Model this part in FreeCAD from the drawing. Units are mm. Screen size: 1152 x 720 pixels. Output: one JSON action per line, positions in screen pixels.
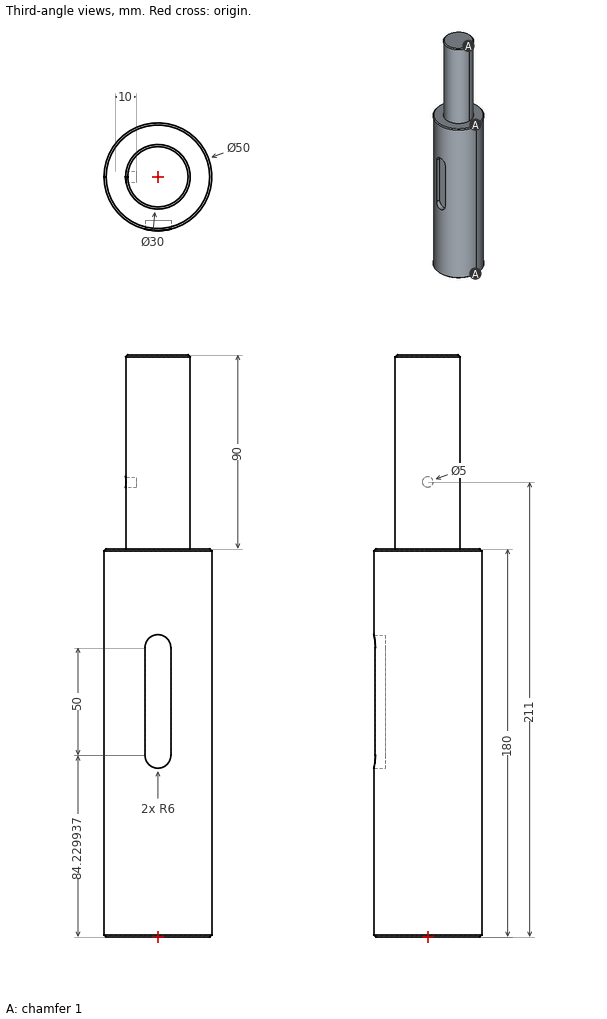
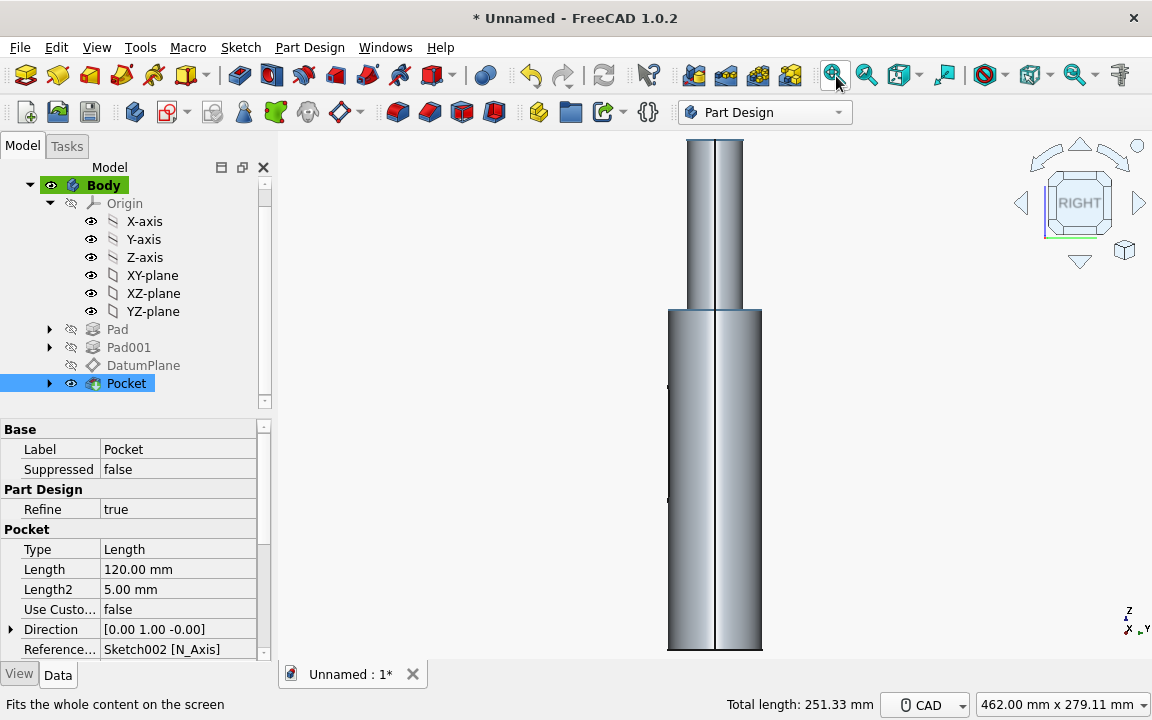
{"action": "key", "text": "5"}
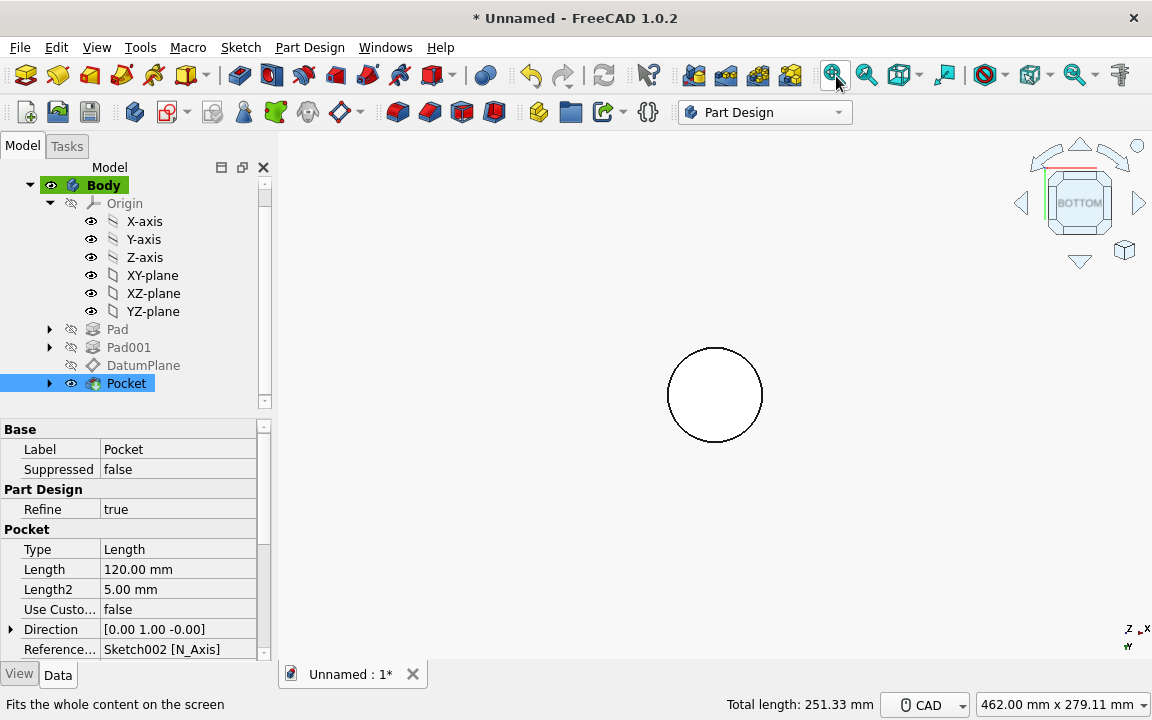
{"action": "key", "text": "v f"}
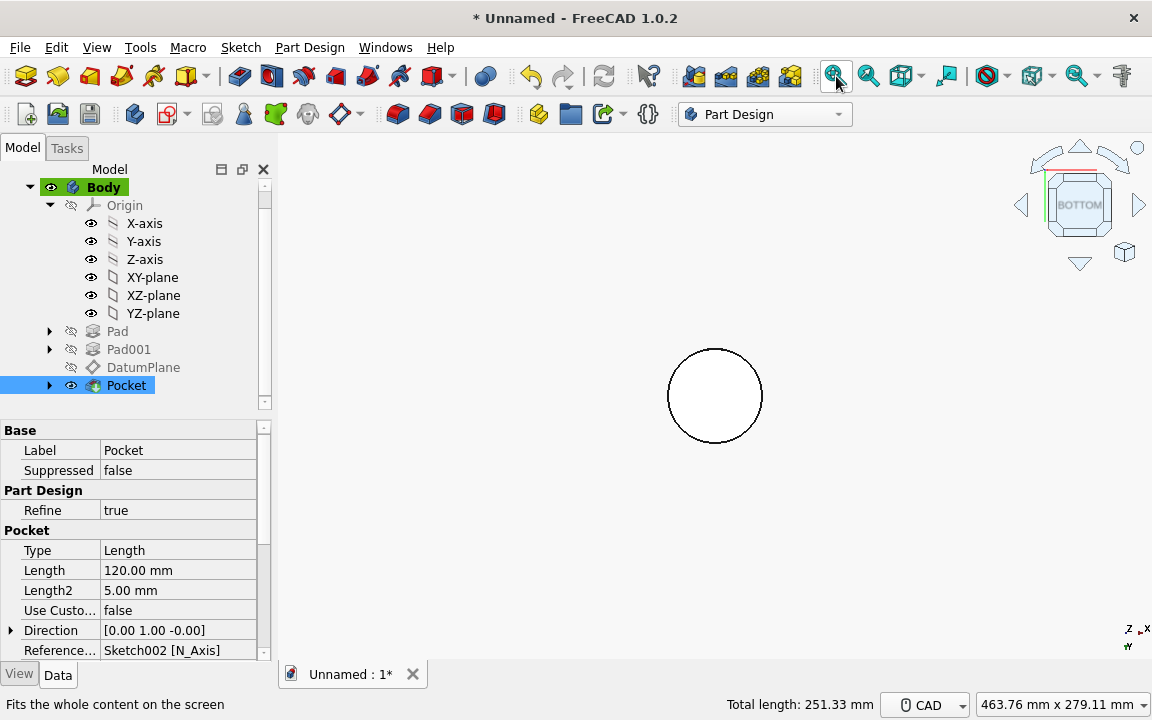
{"action": "left_click", "coordinate": [668, 395], "text": "ctrl"}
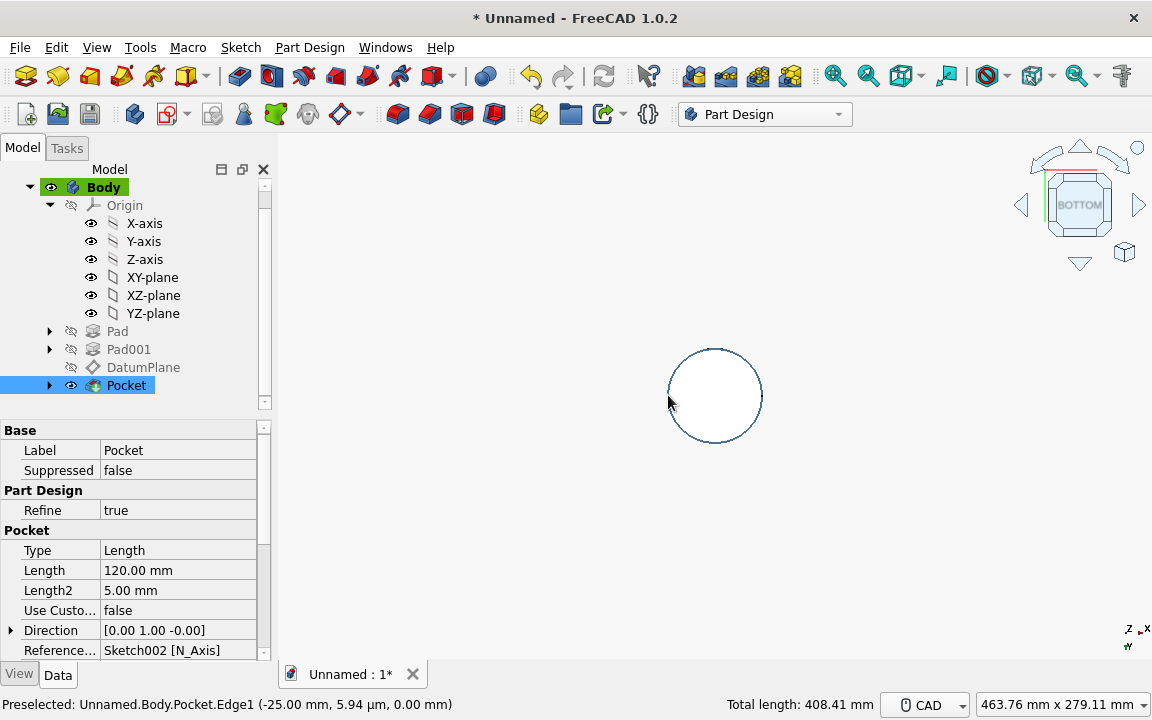
{"action": "left_click", "coordinate": [430, 114]}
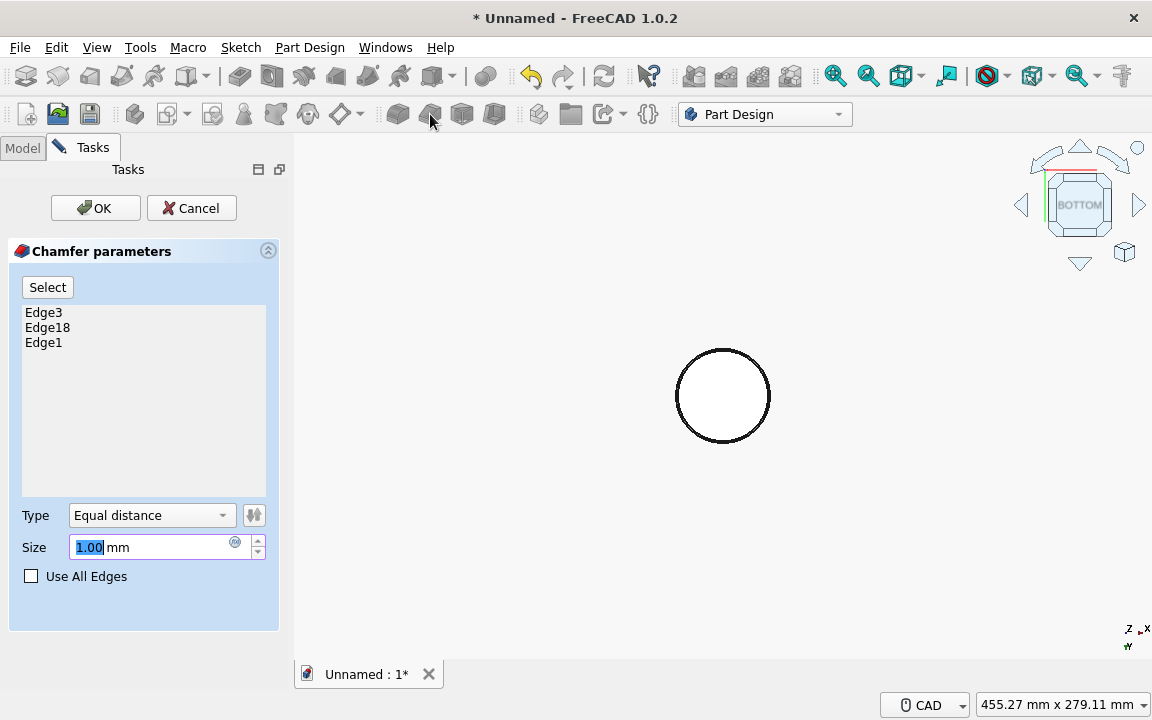
{"action": "type", "text": "1"}
{"action": "key", "text": "Tab"}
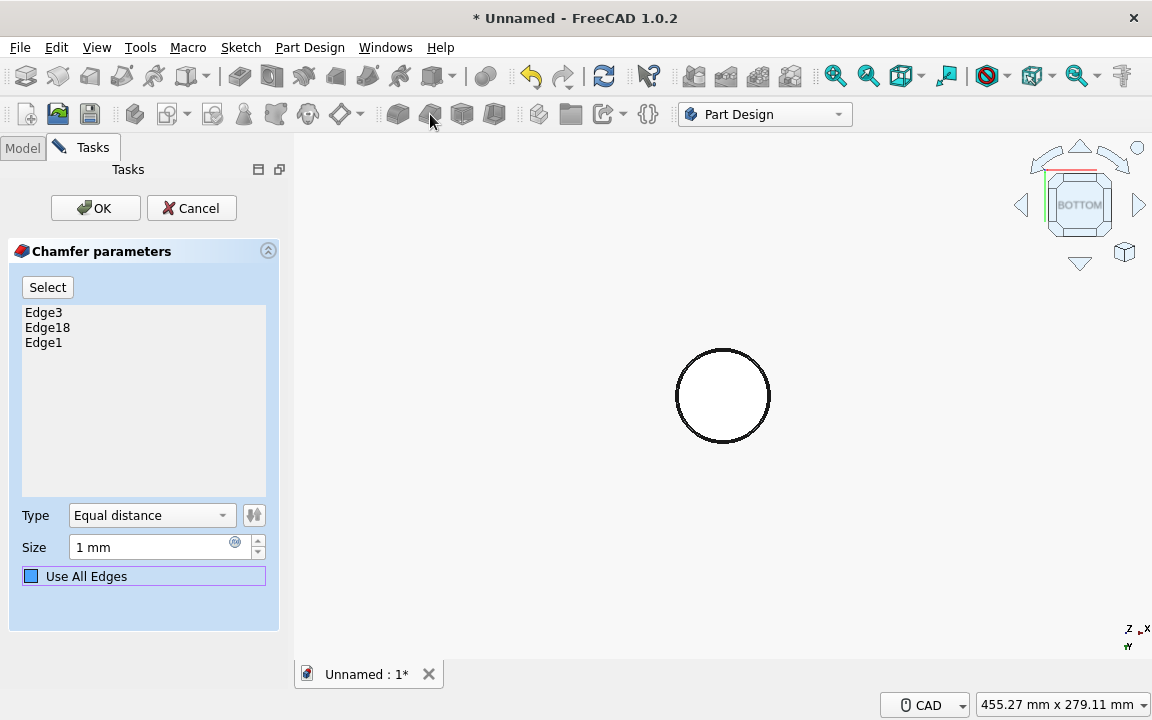
{"action": "left_click", "coordinate": [96, 208]}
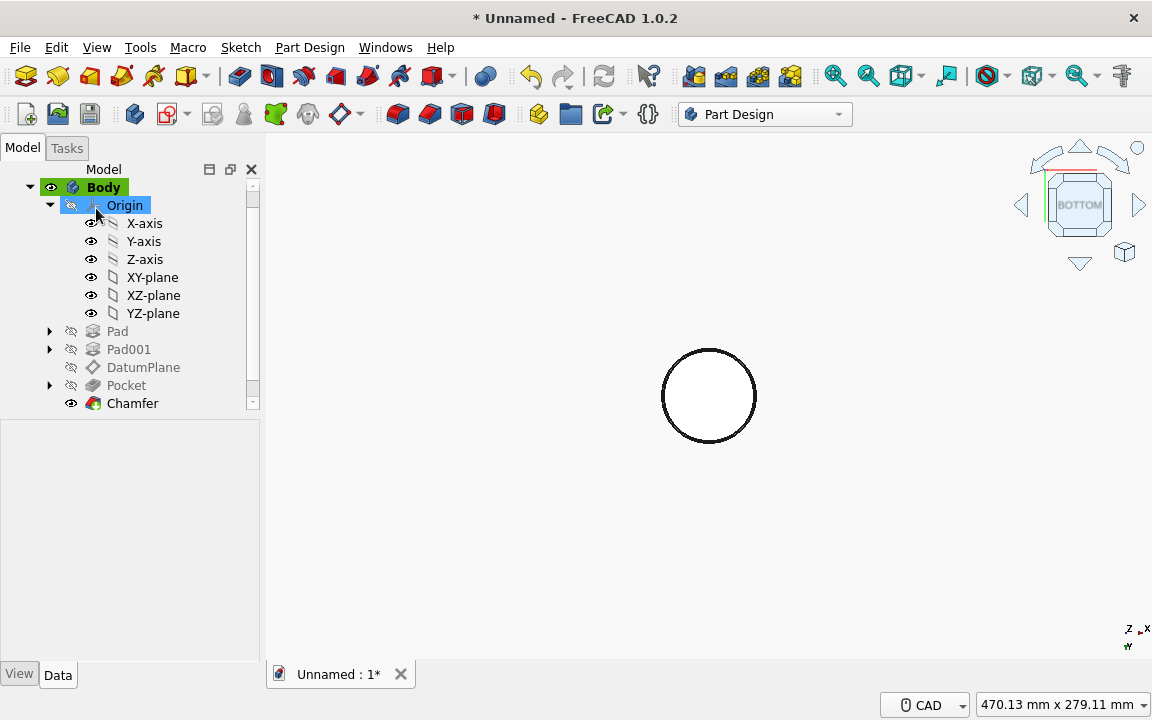
{"action": "key", "text": "v f"}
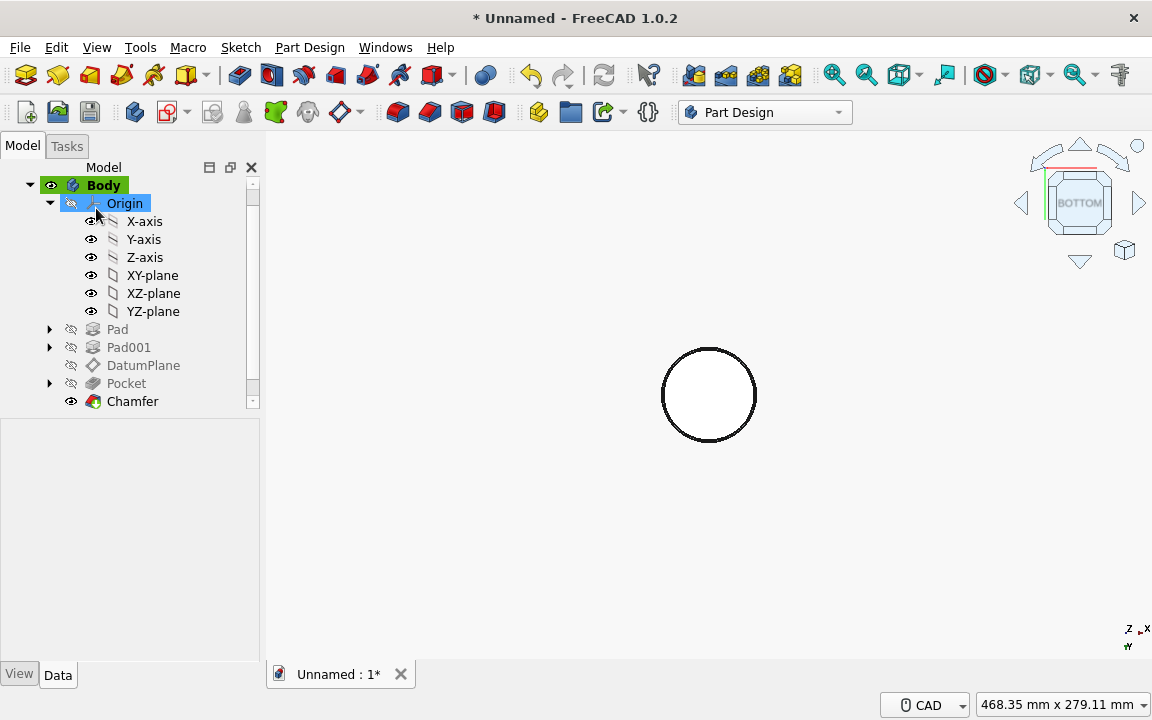
{"action": "left_click", "coordinate": [136, 311]}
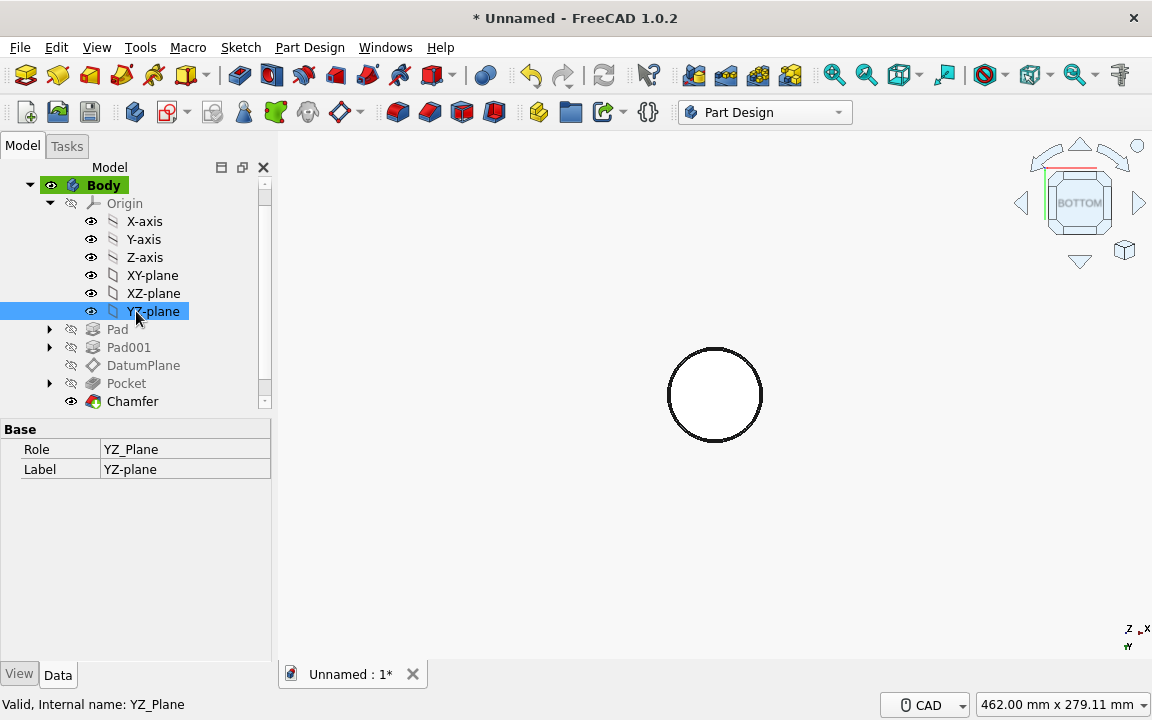
{"action": "left_click", "coordinate": [340, 112]}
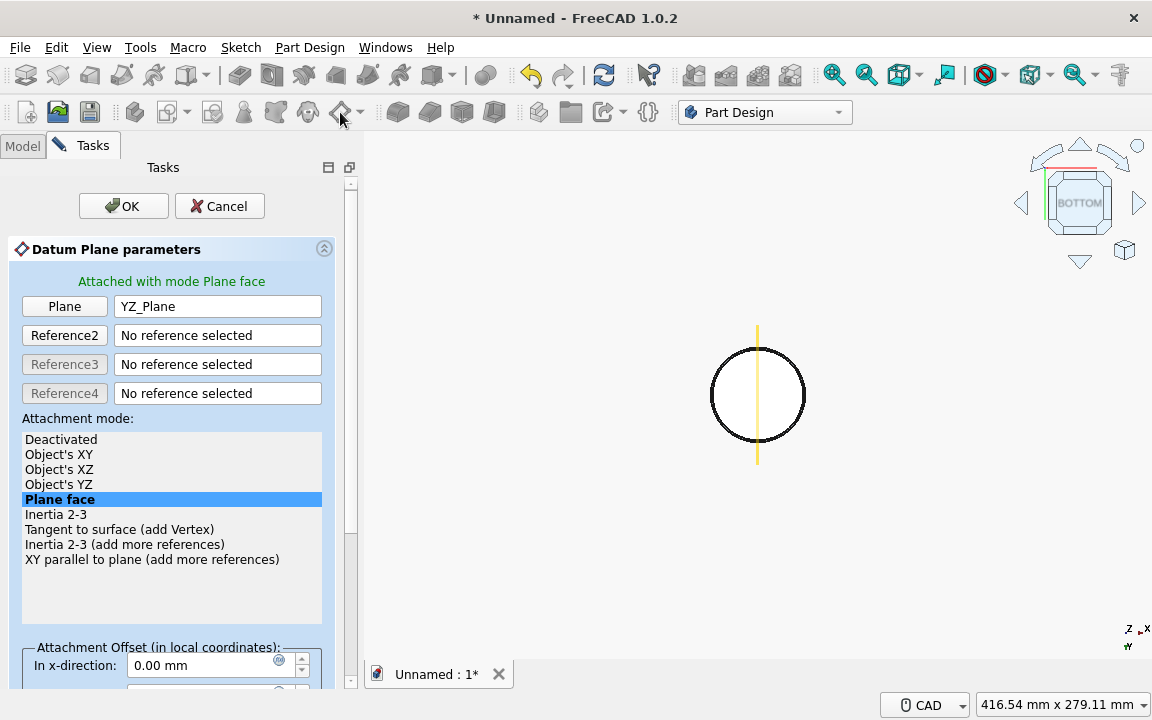
{"action": "scroll", "coordinate": [351, 432], "scroll_direction": "down", "scroll_amount": 2}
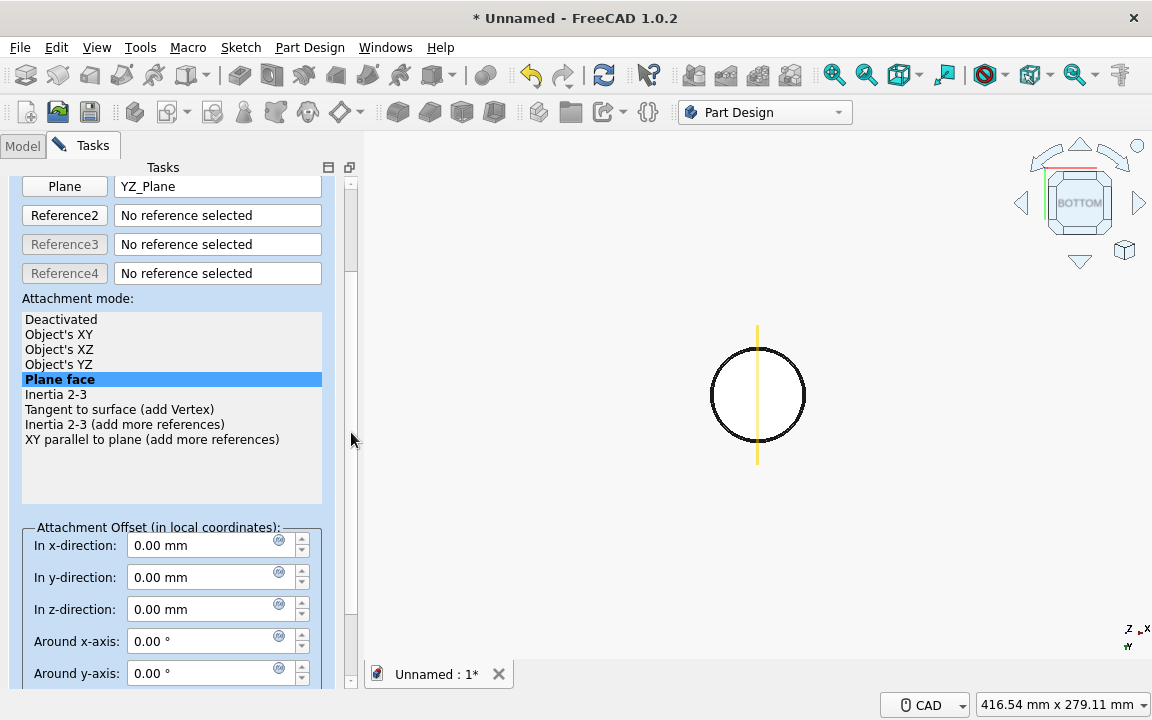
{"action": "triple_click", "coordinate": [210, 609]}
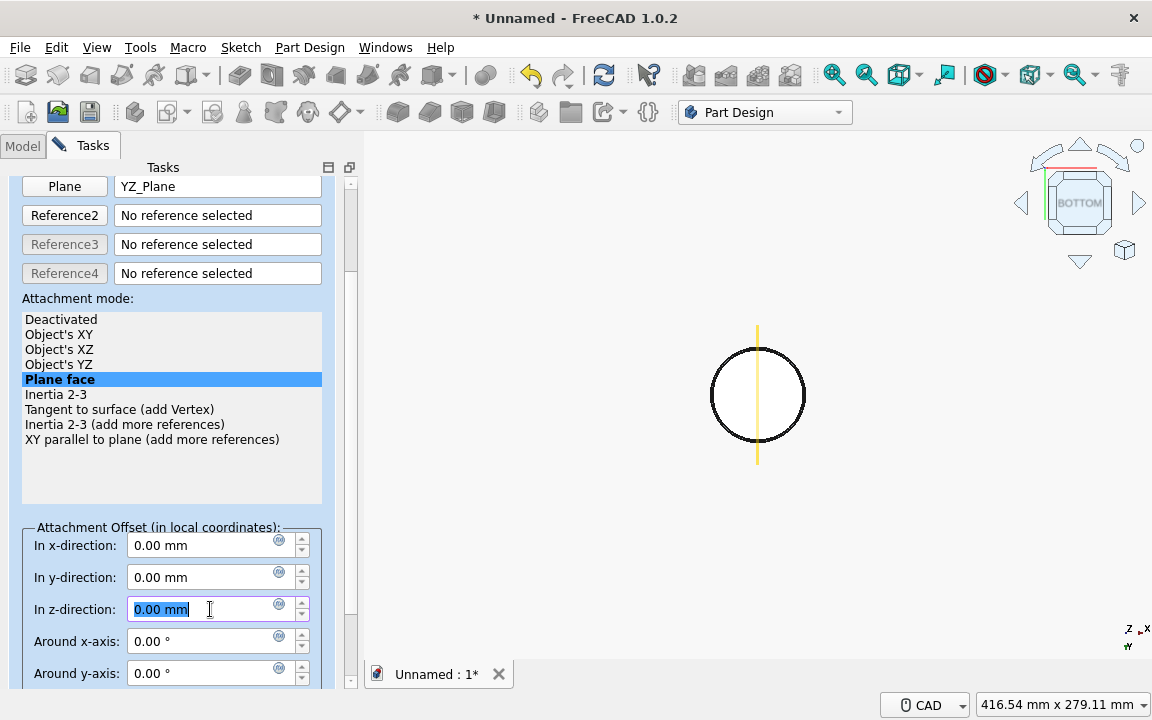
{"action": "type", "text": "-10"}
{"action": "key", "text": "Tab"}